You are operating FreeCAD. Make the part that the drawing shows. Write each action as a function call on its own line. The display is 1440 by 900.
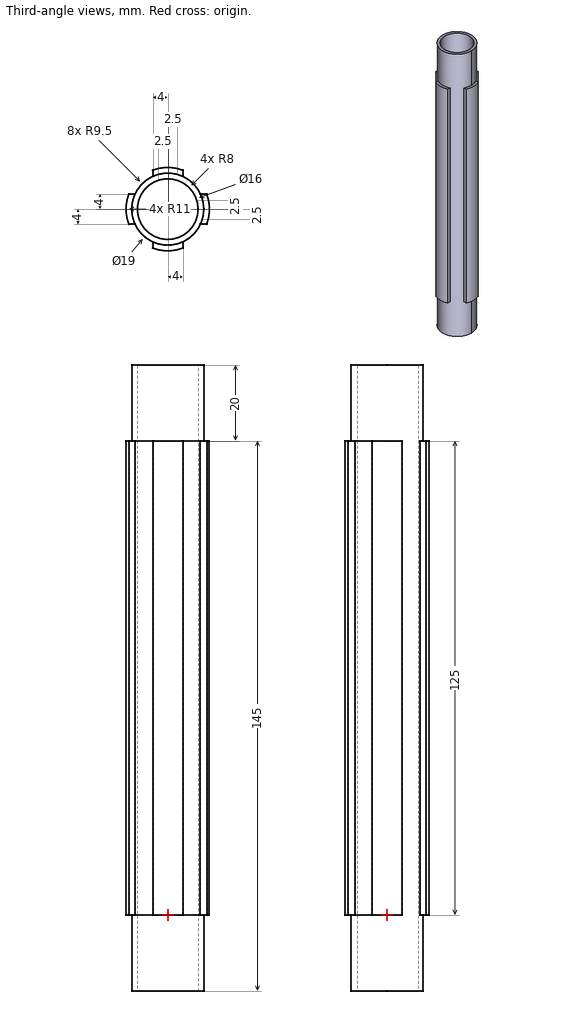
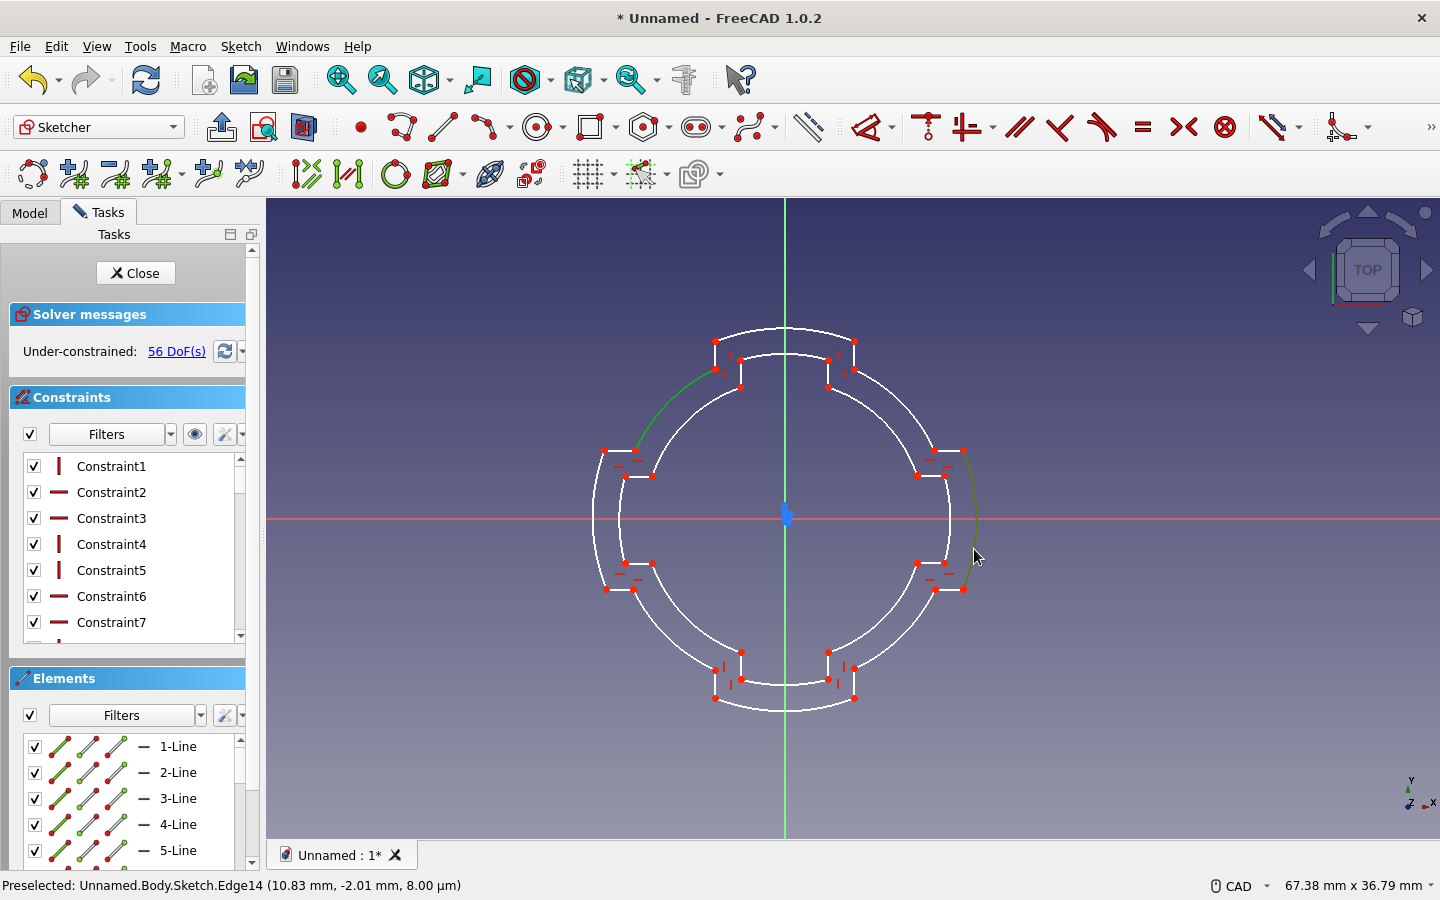
click(926, 128)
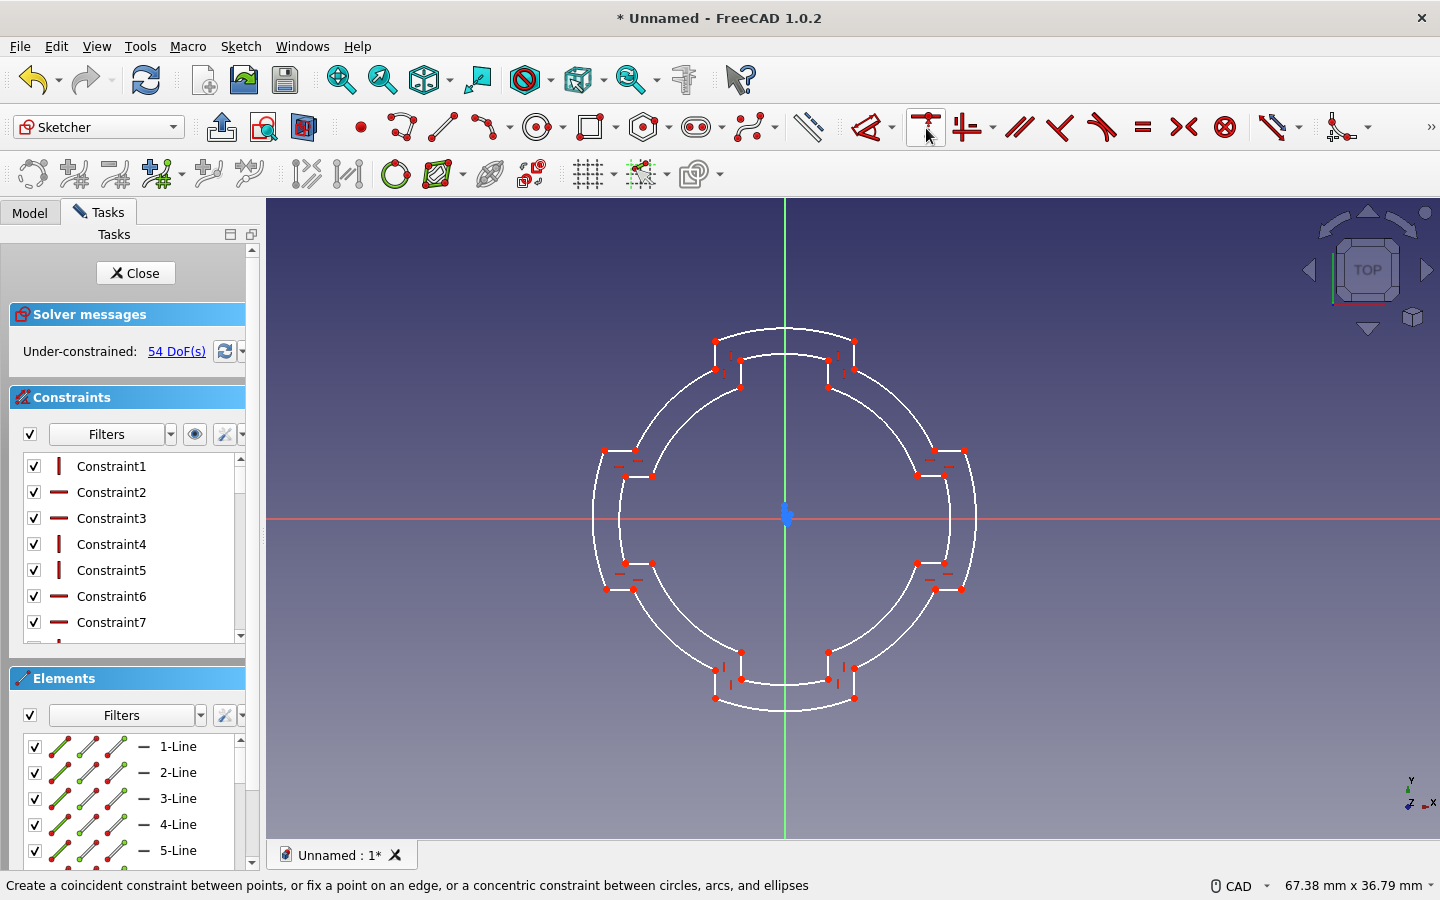
click(686, 387)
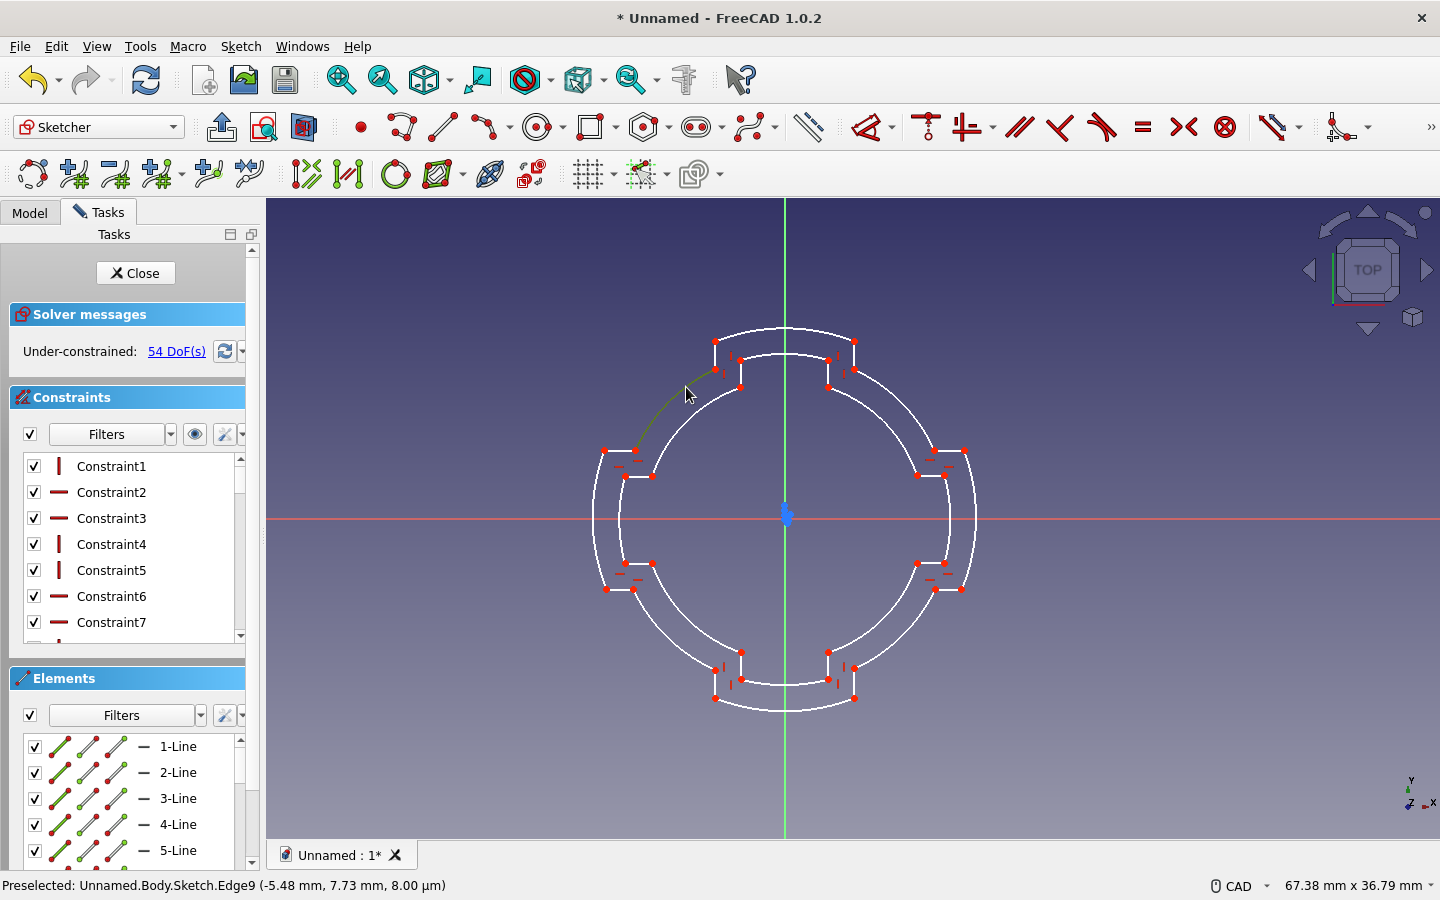
click(917, 421)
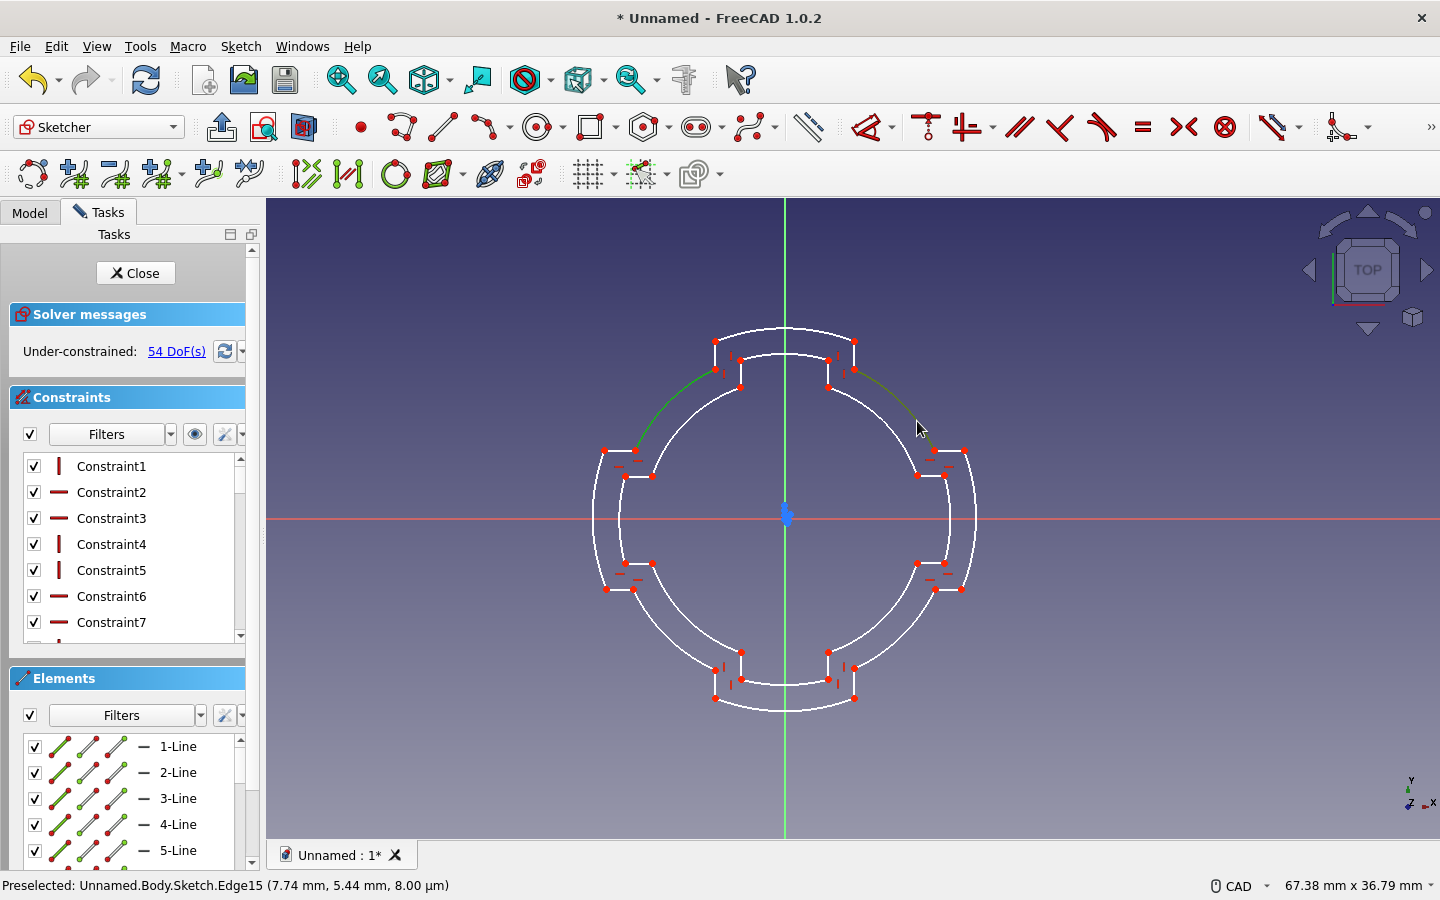
click(926, 128)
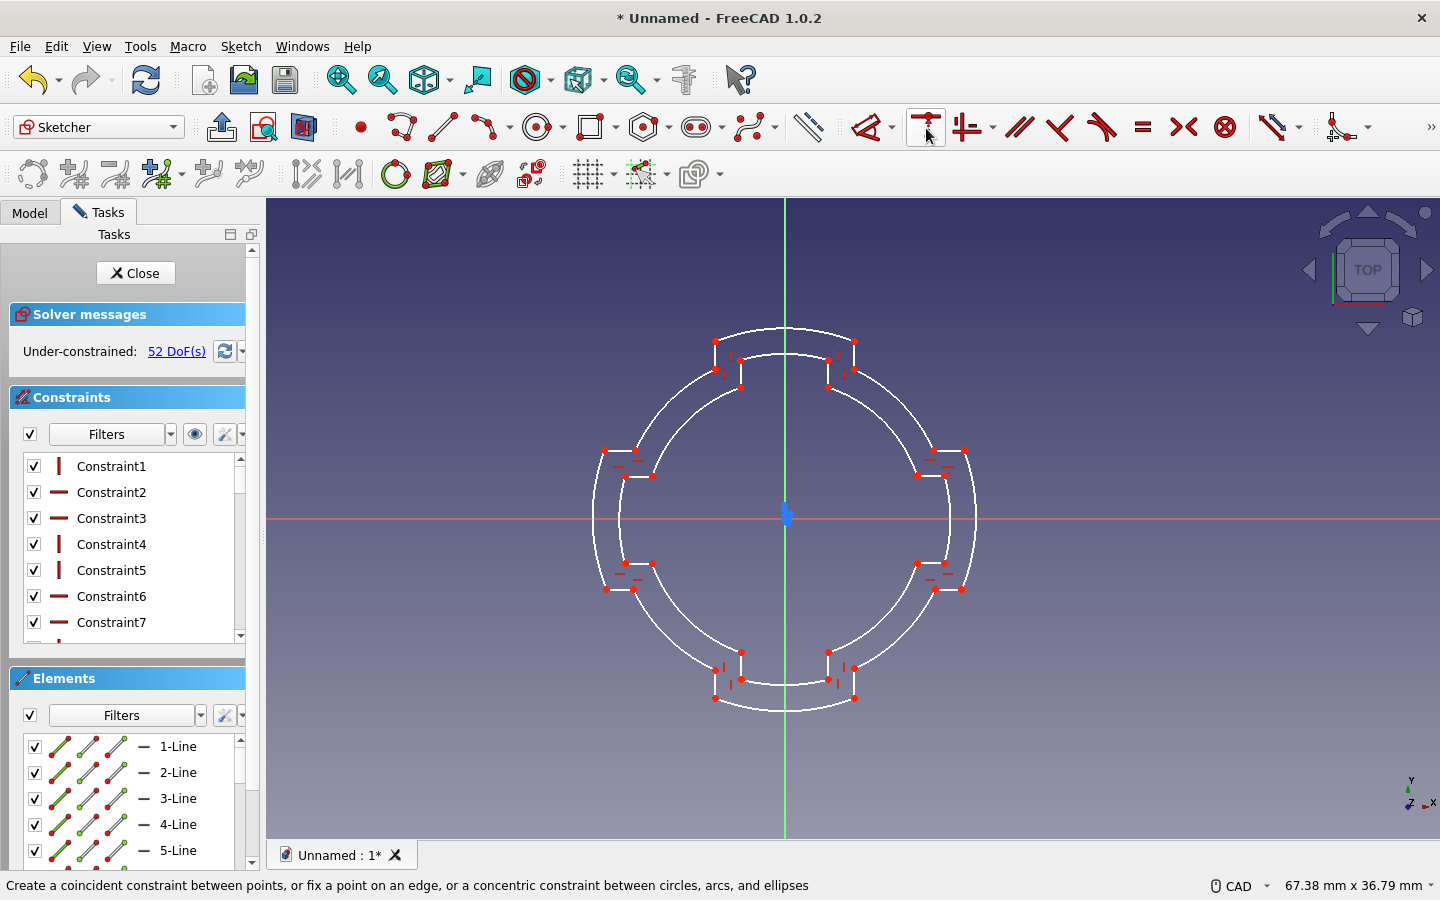
click(686, 387)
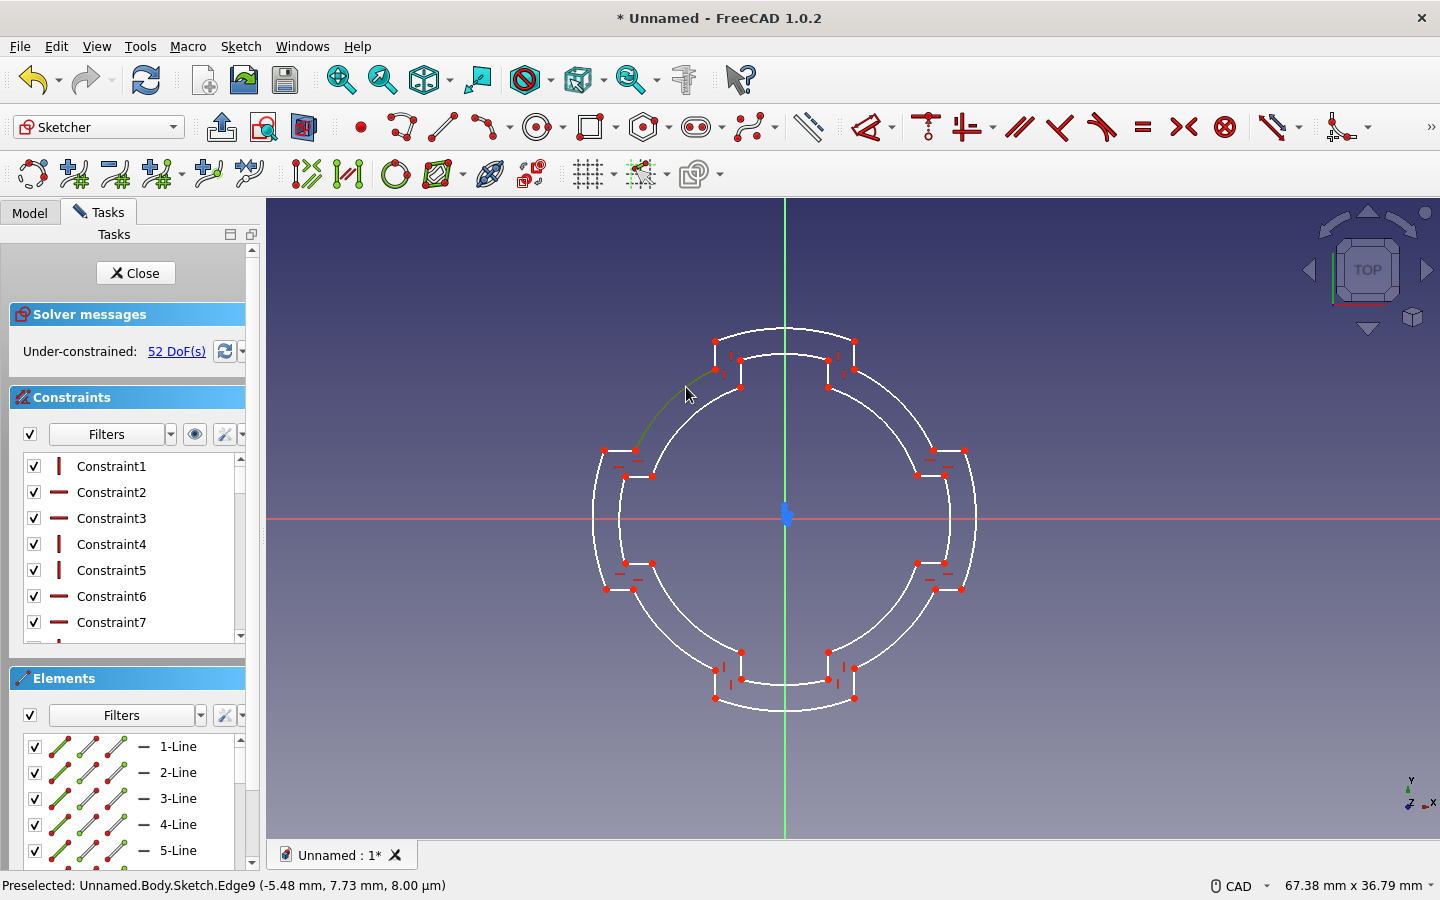
click(813, 330)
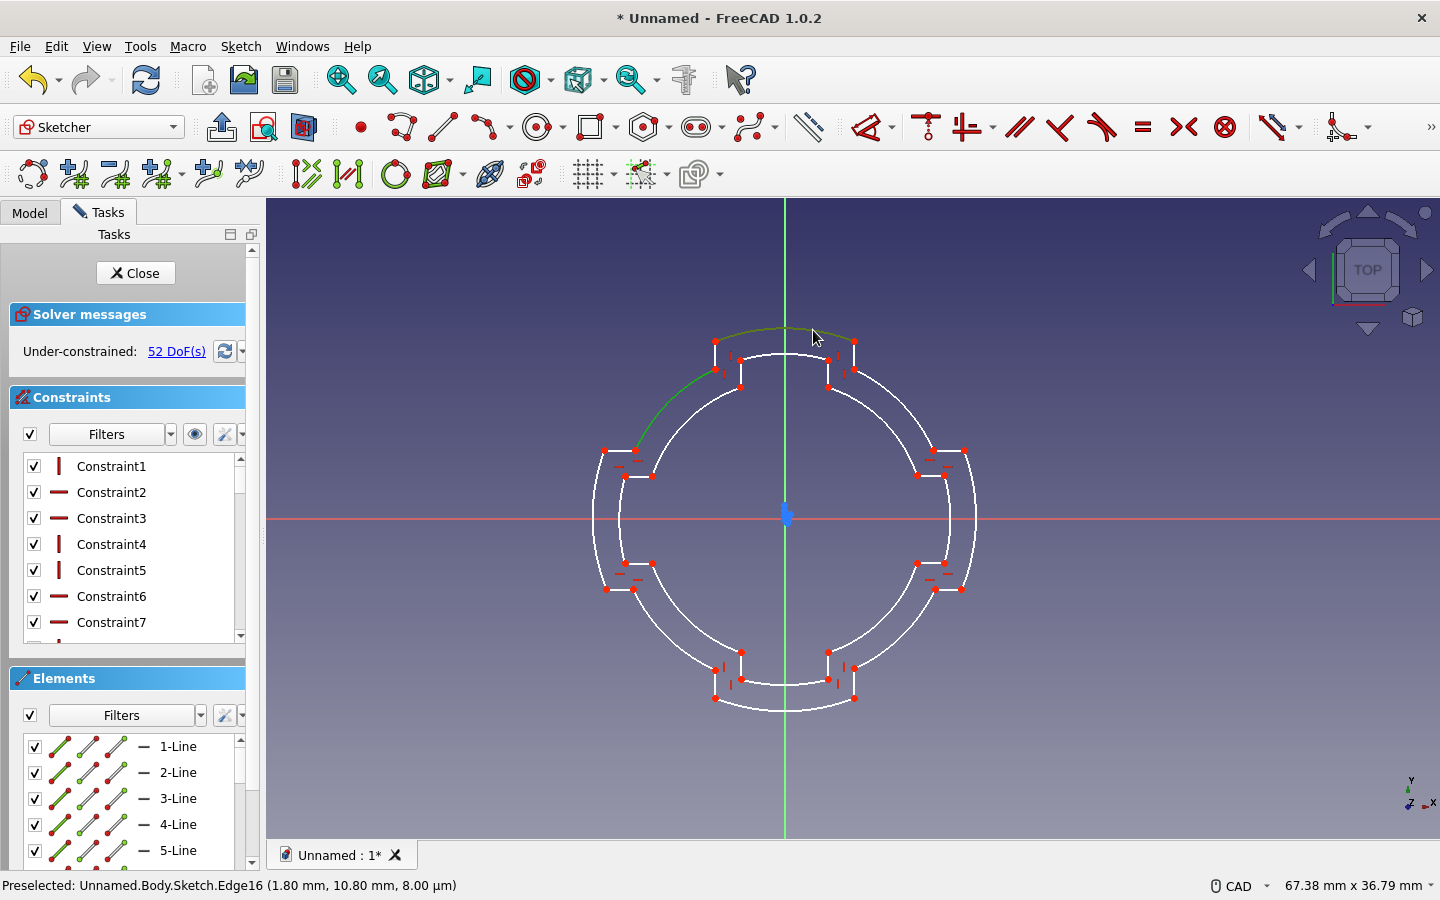
click(926, 128)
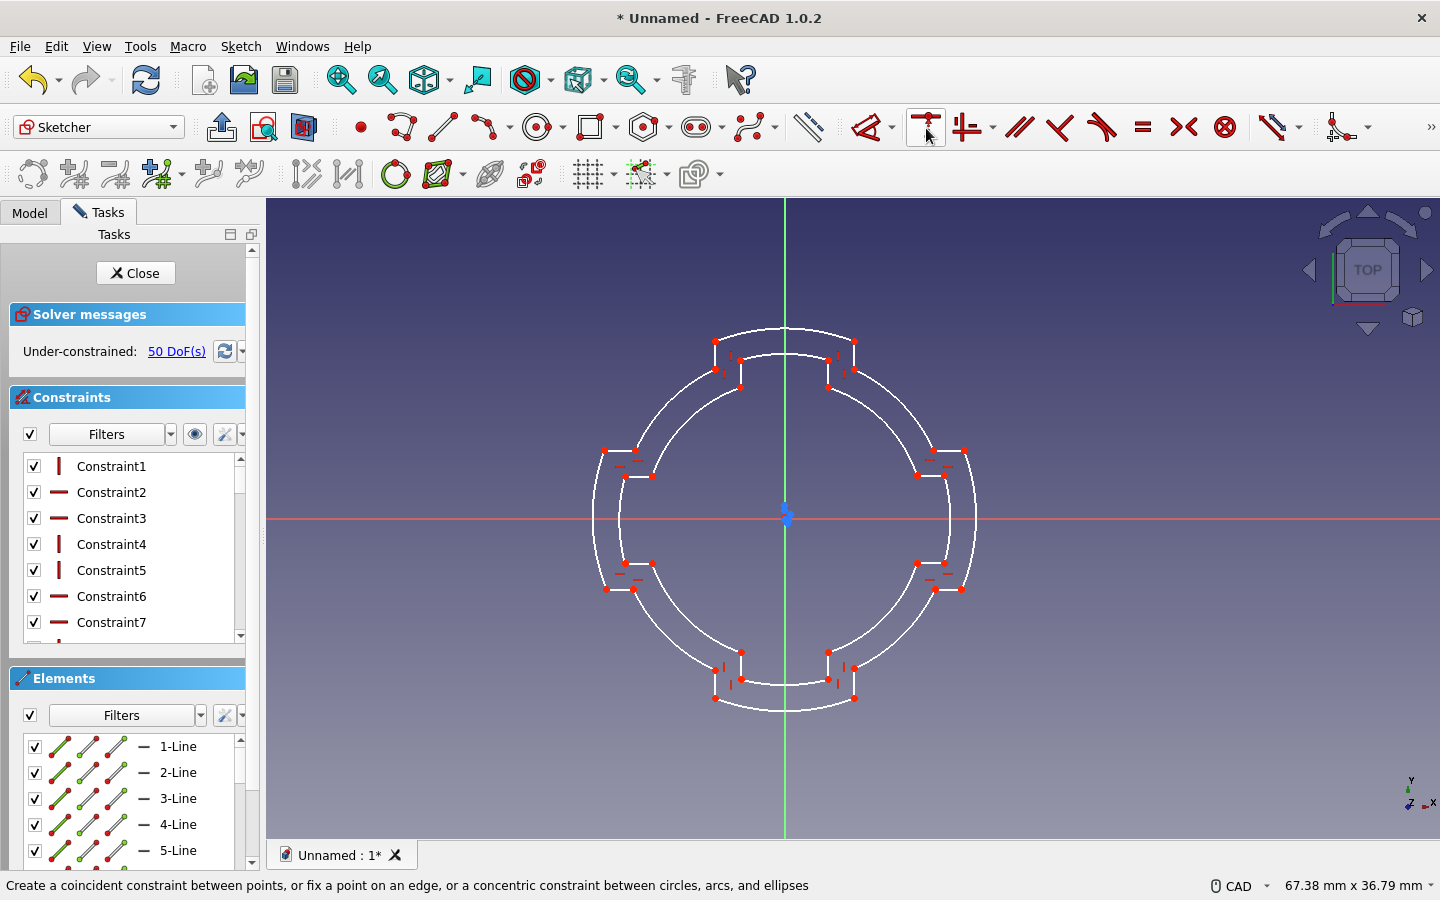
click(686, 387)